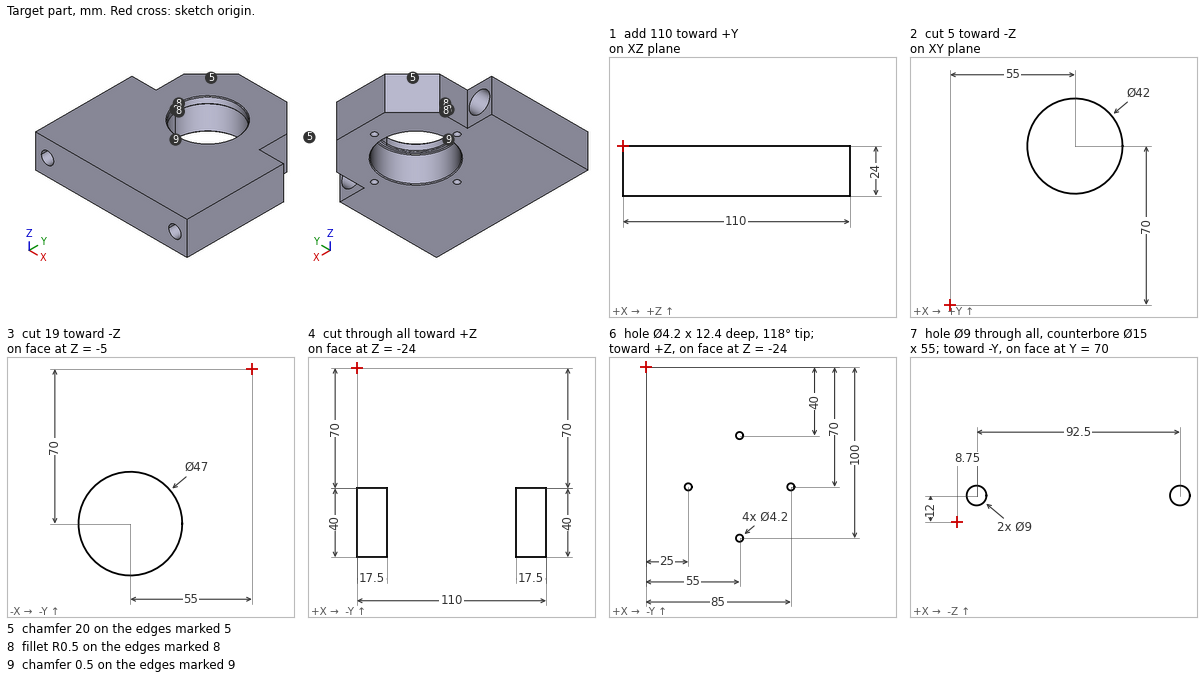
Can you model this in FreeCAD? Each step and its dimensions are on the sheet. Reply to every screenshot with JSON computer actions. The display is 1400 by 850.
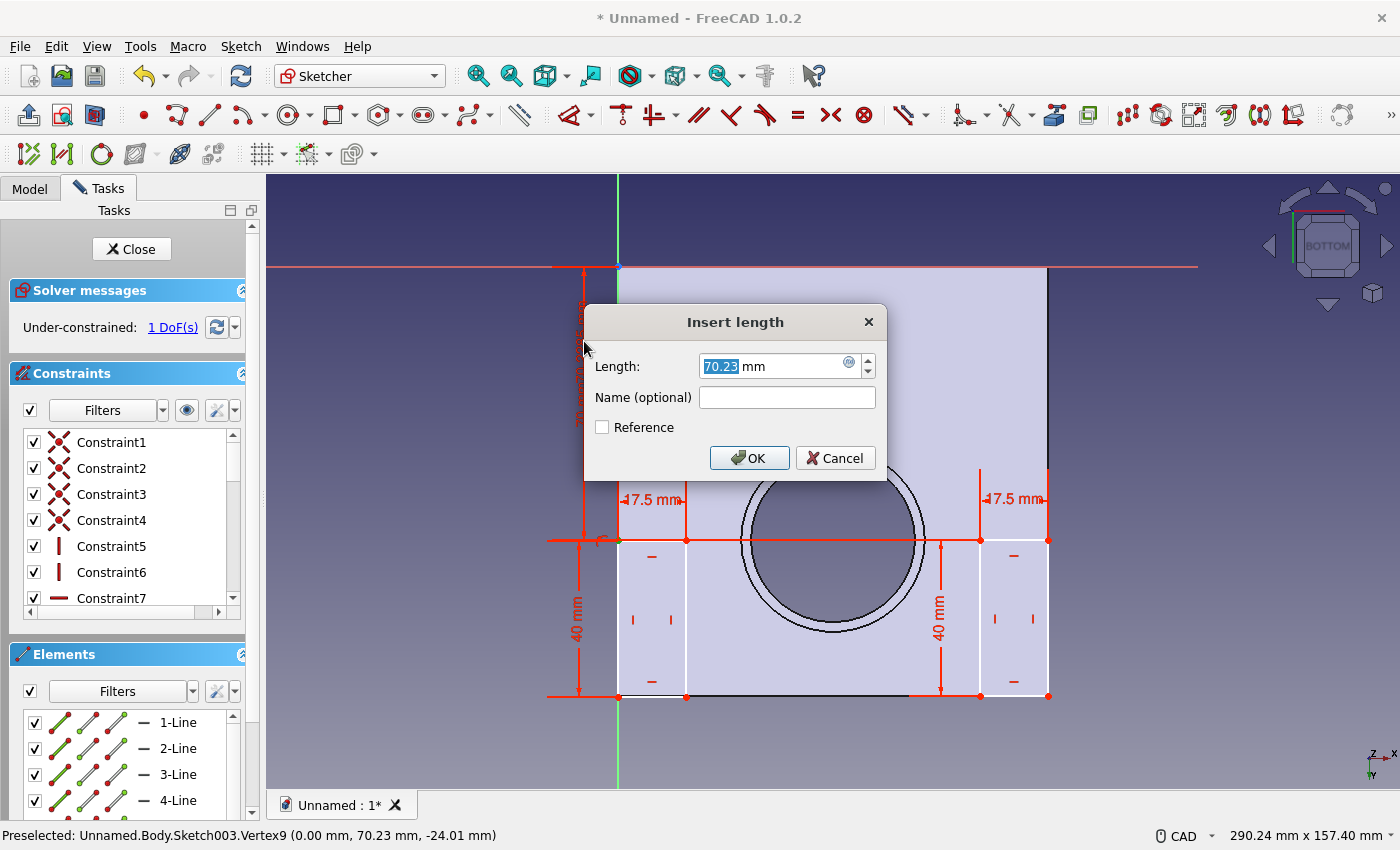
{"action": "type", "text": "70"}
{"action": "key", "text": "Return"}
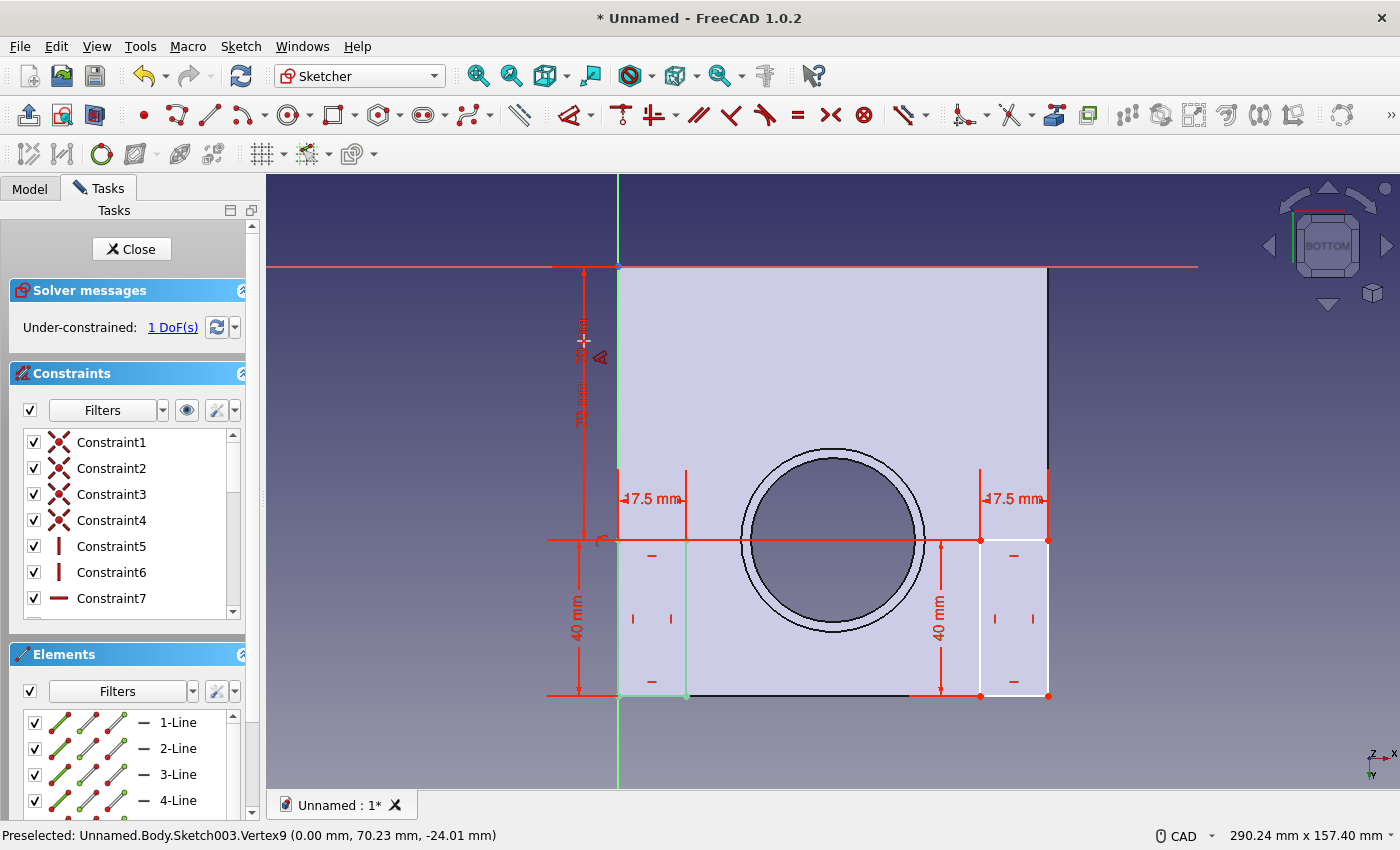
{"action": "left_click", "coordinate": [1048, 696]}
{"action": "left_click", "coordinate": [833, 233]}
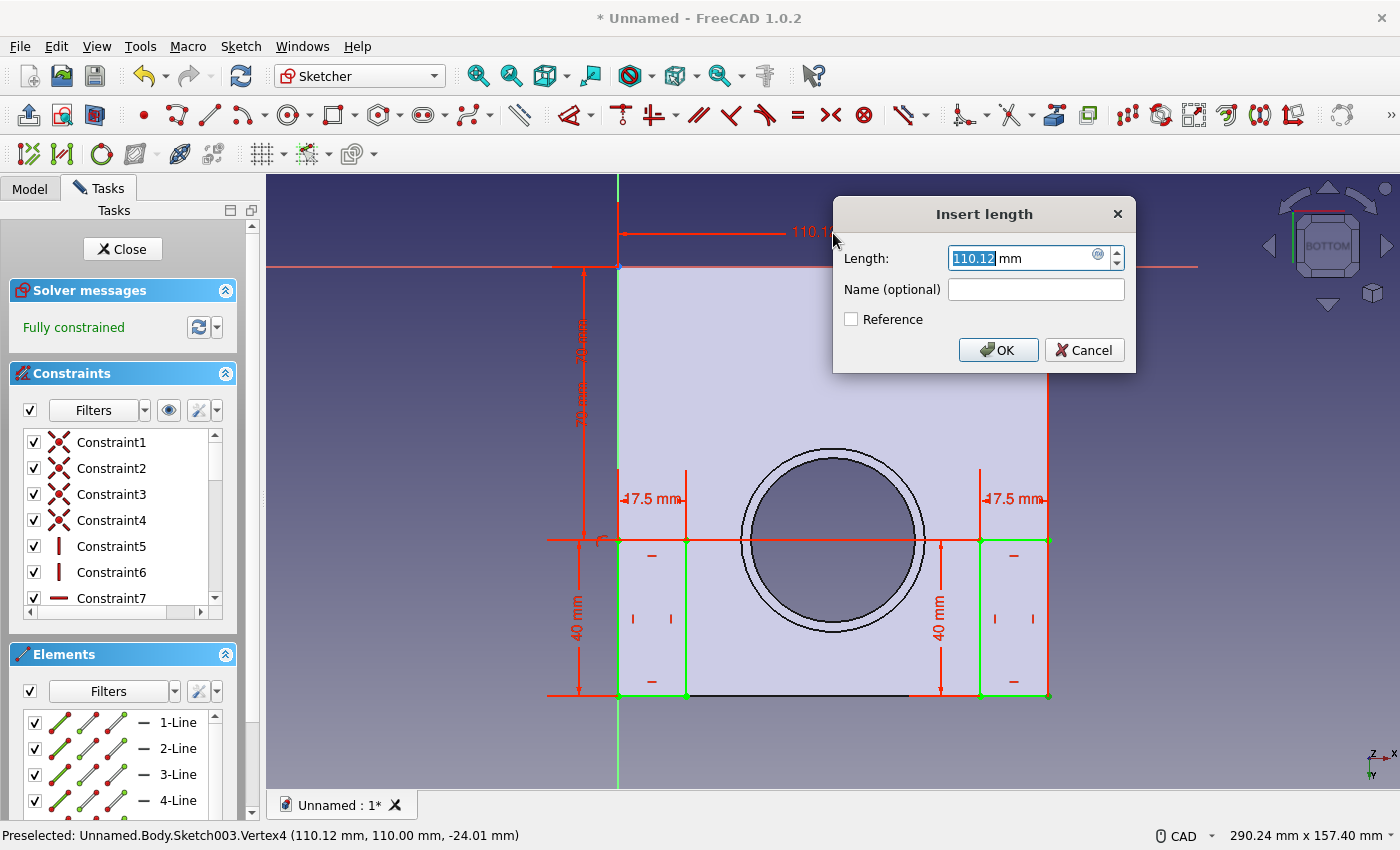
{"action": "type", "text": "110"}
{"action": "key", "text": "Return"}
{"action": "key", "text": "Escape"}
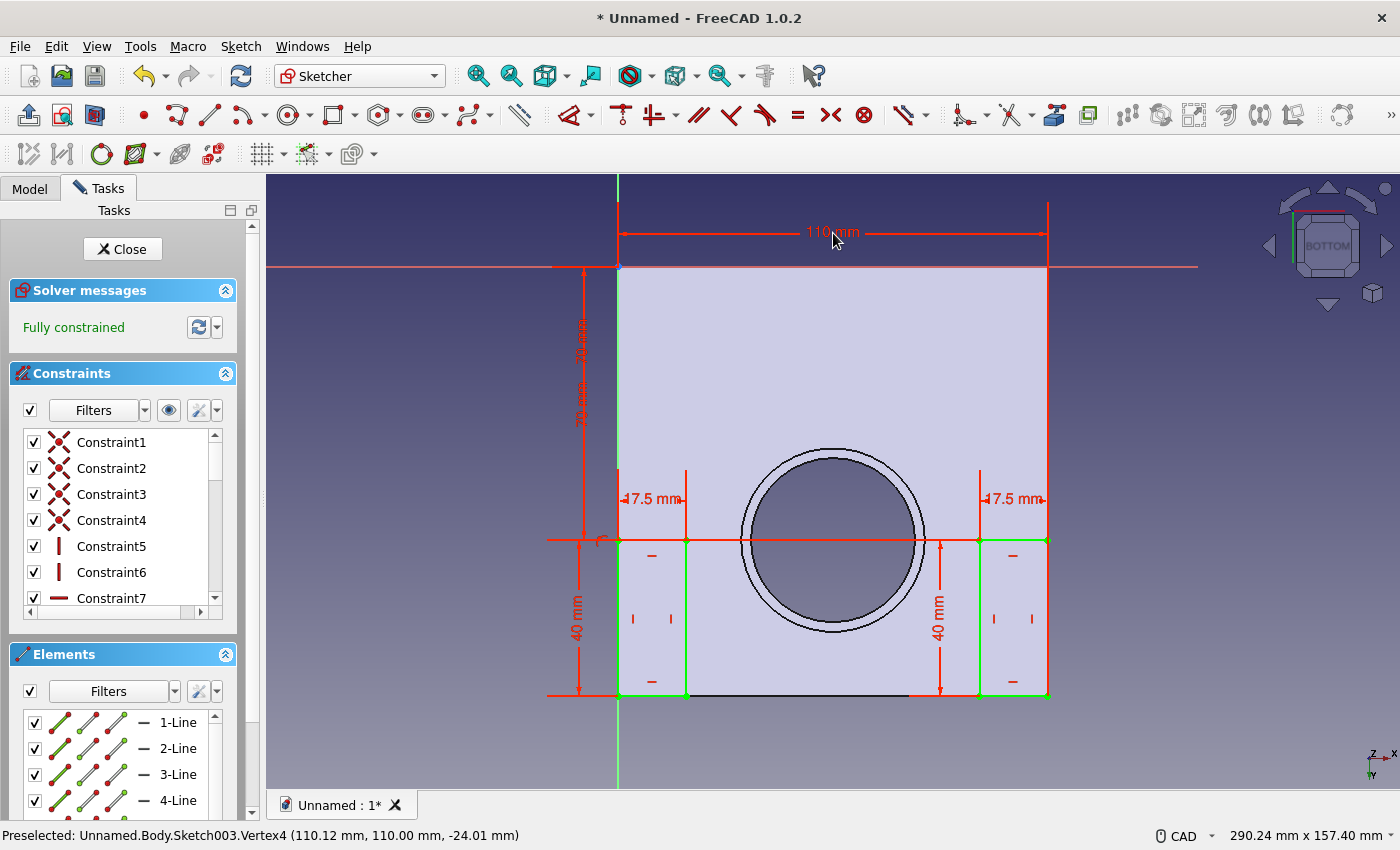
{"action": "left_click", "coordinate": [123, 249]}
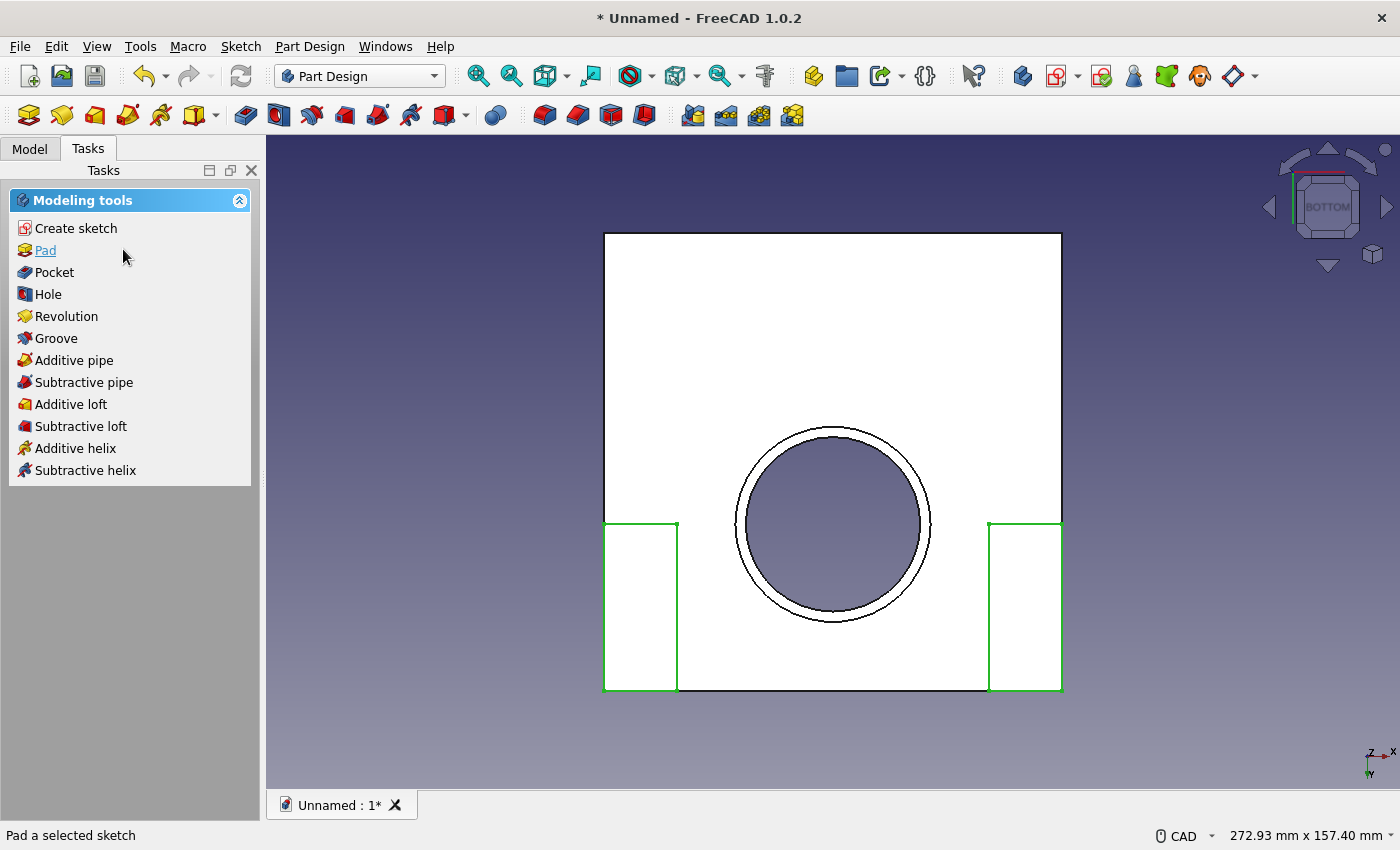
{"action": "left_click", "coordinate": [246, 116]}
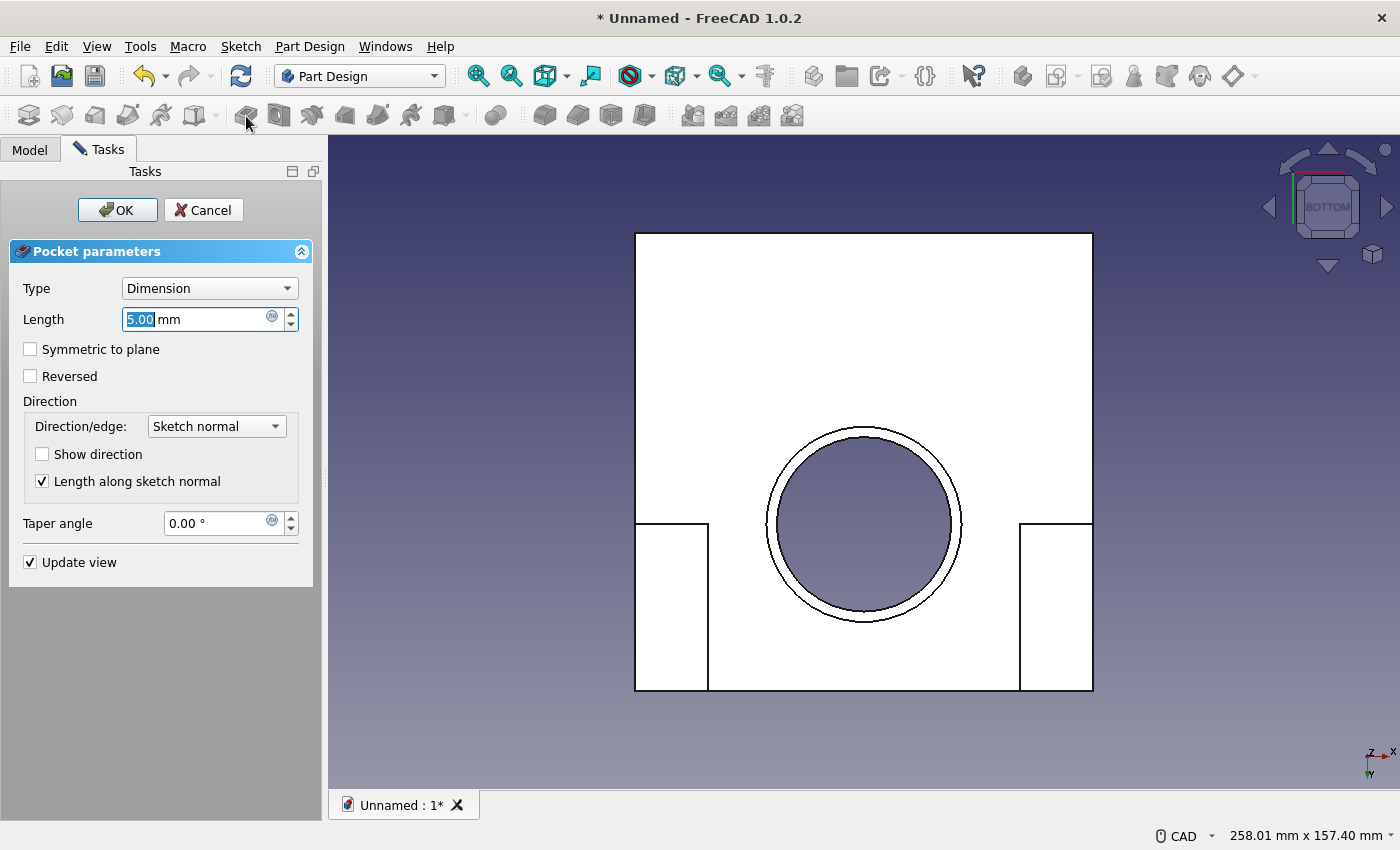
{"action": "left_click", "coordinate": [210, 288]}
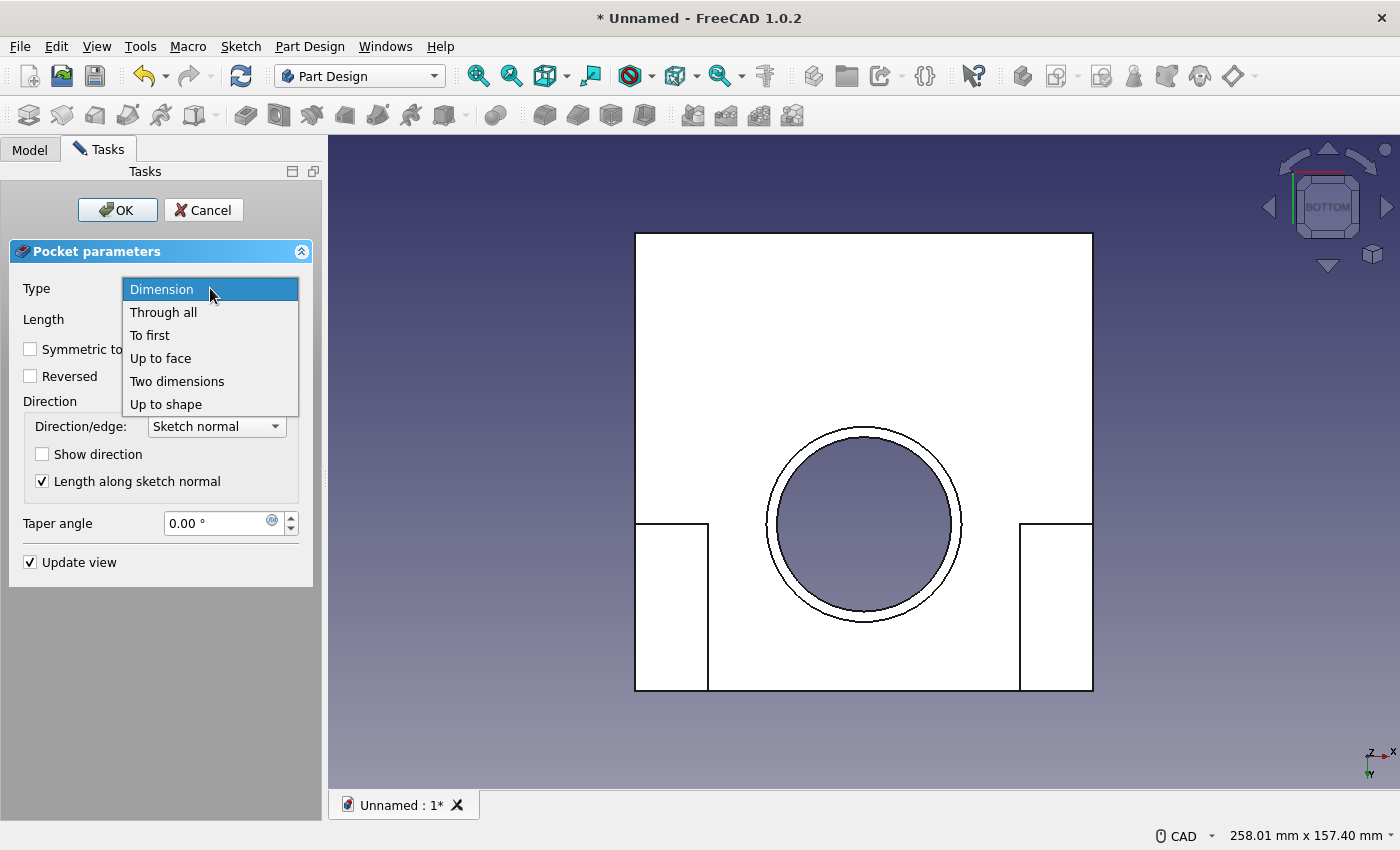
{"action": "left_click", "coordinate": [208, 312]}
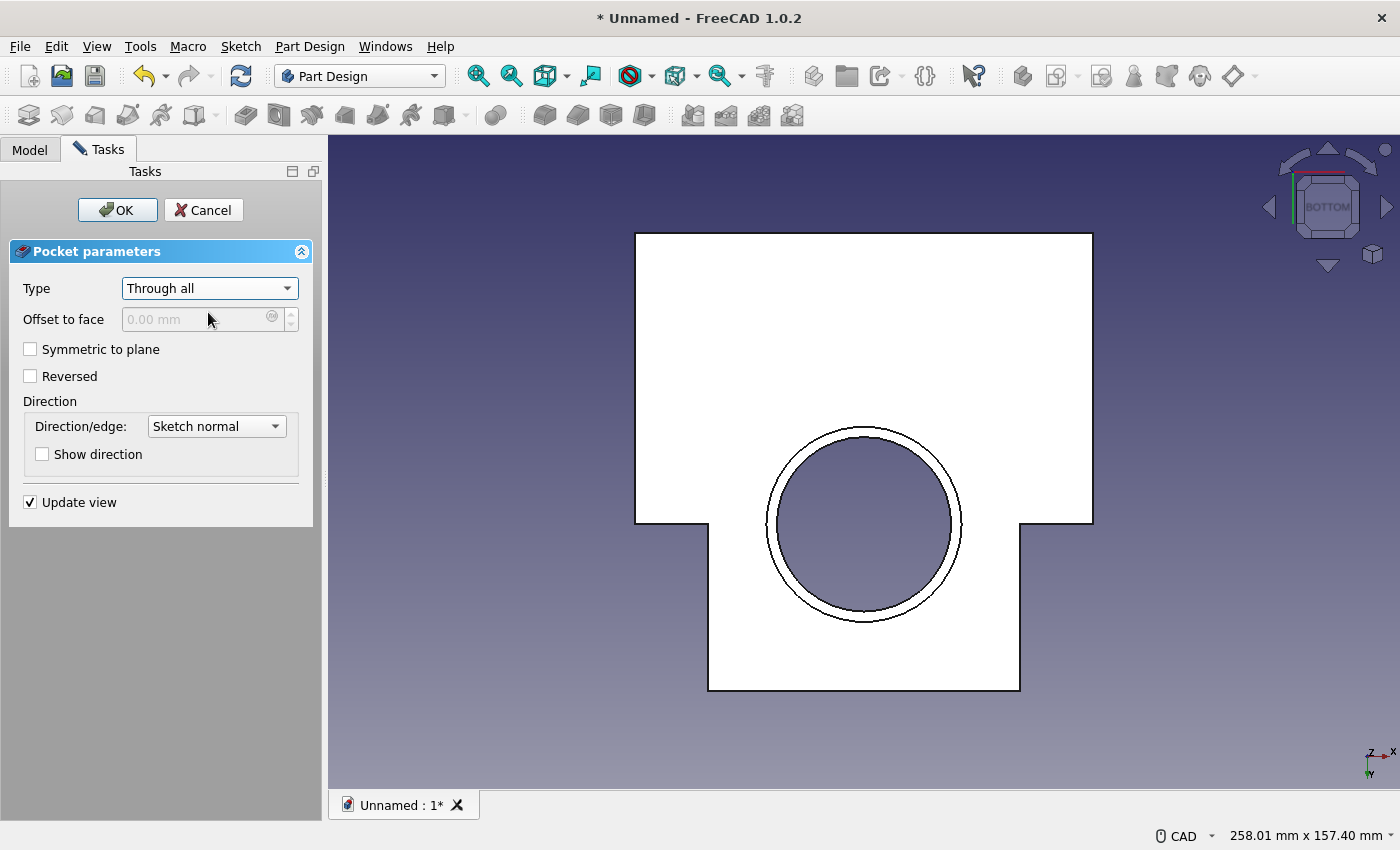
{"action": "left_click", "coordinate": [118, 210]}